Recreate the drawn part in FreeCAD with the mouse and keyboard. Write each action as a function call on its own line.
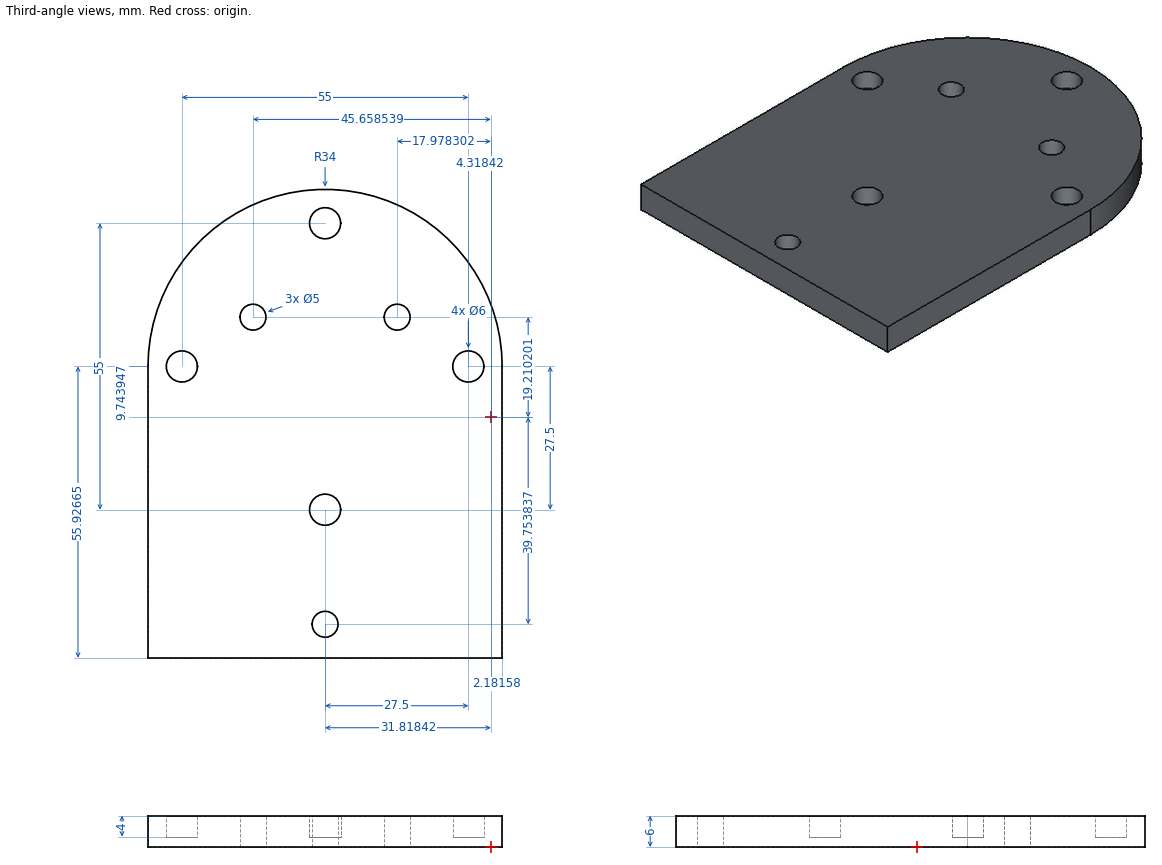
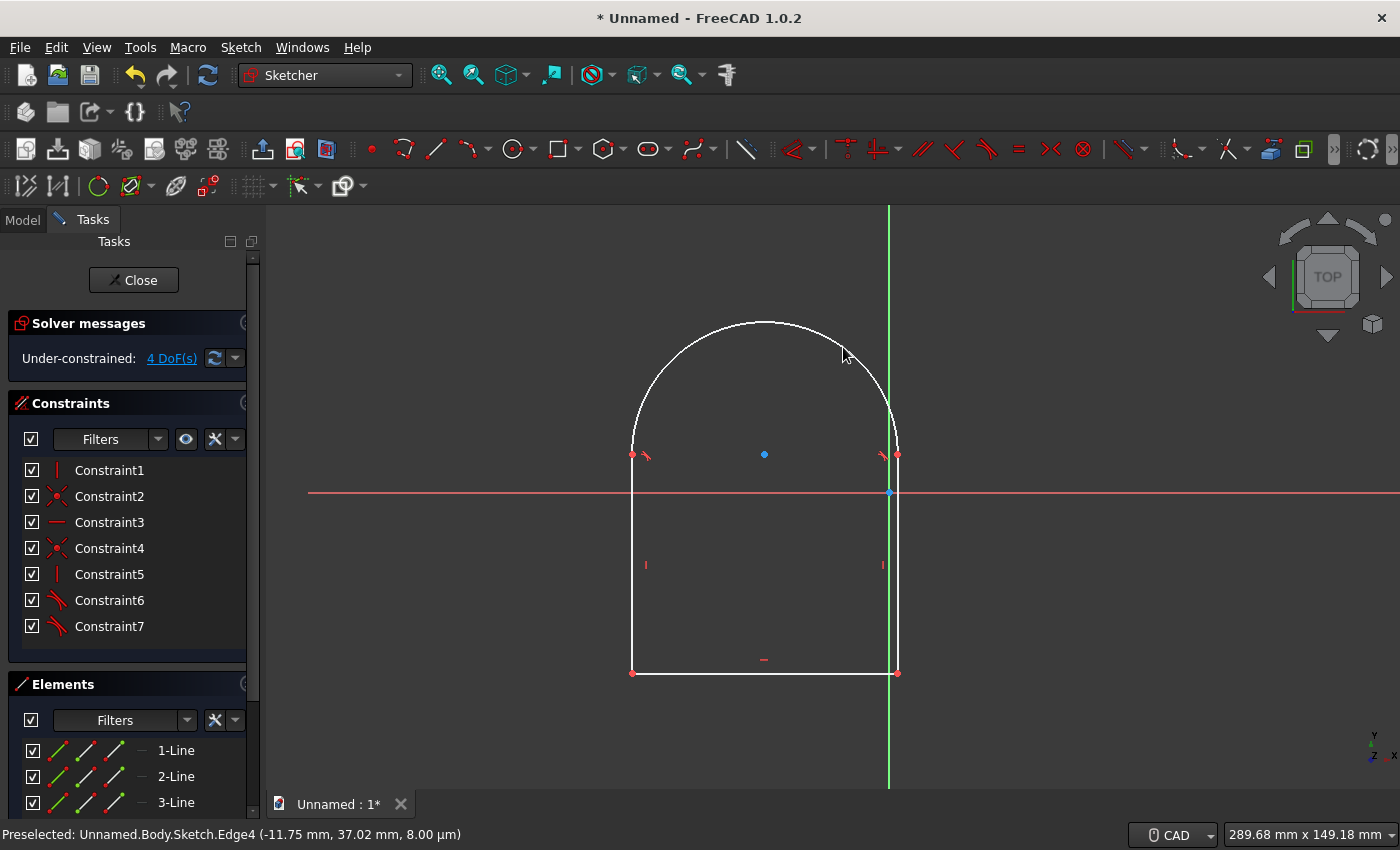
click(843, 347)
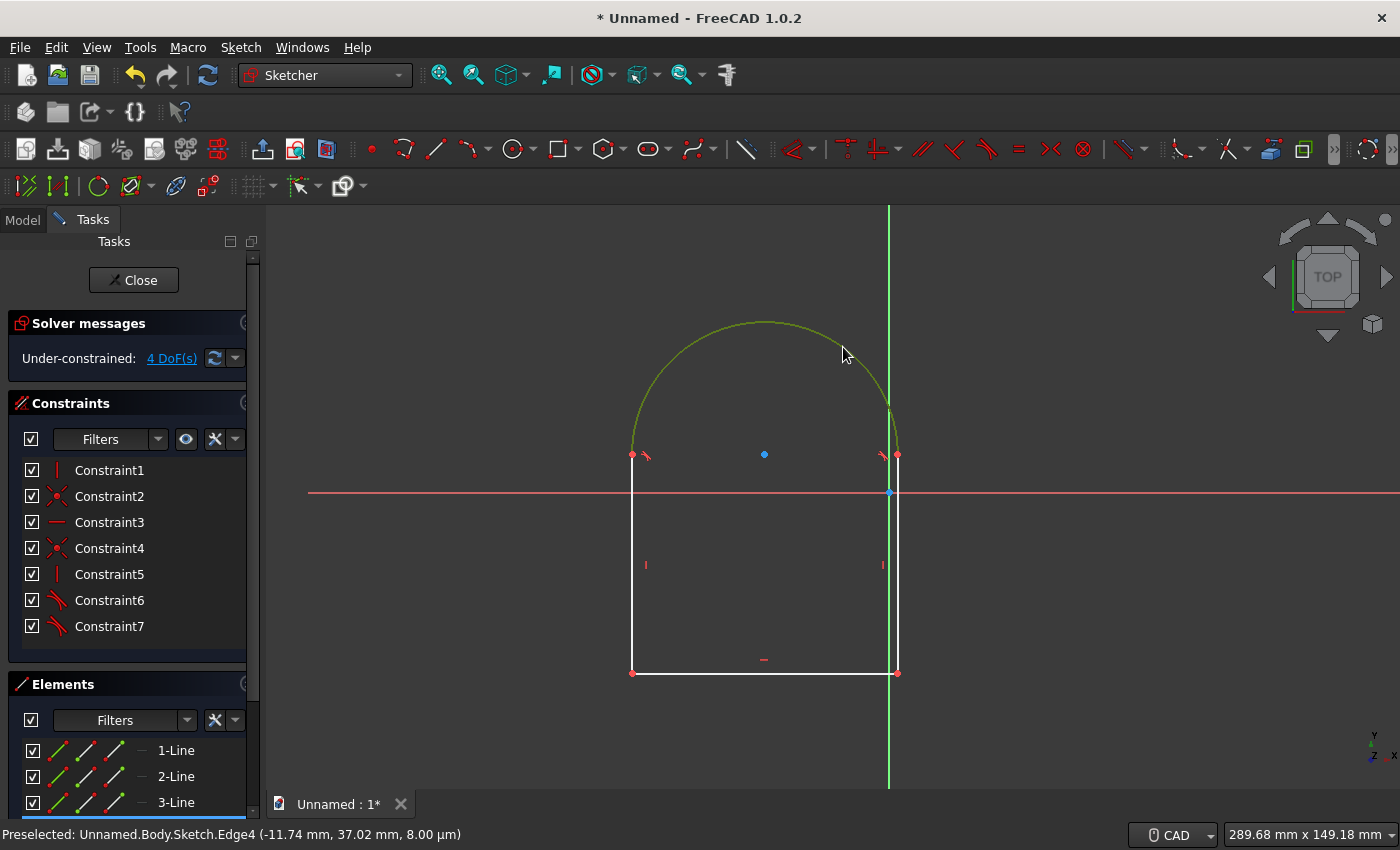
click(814, 150)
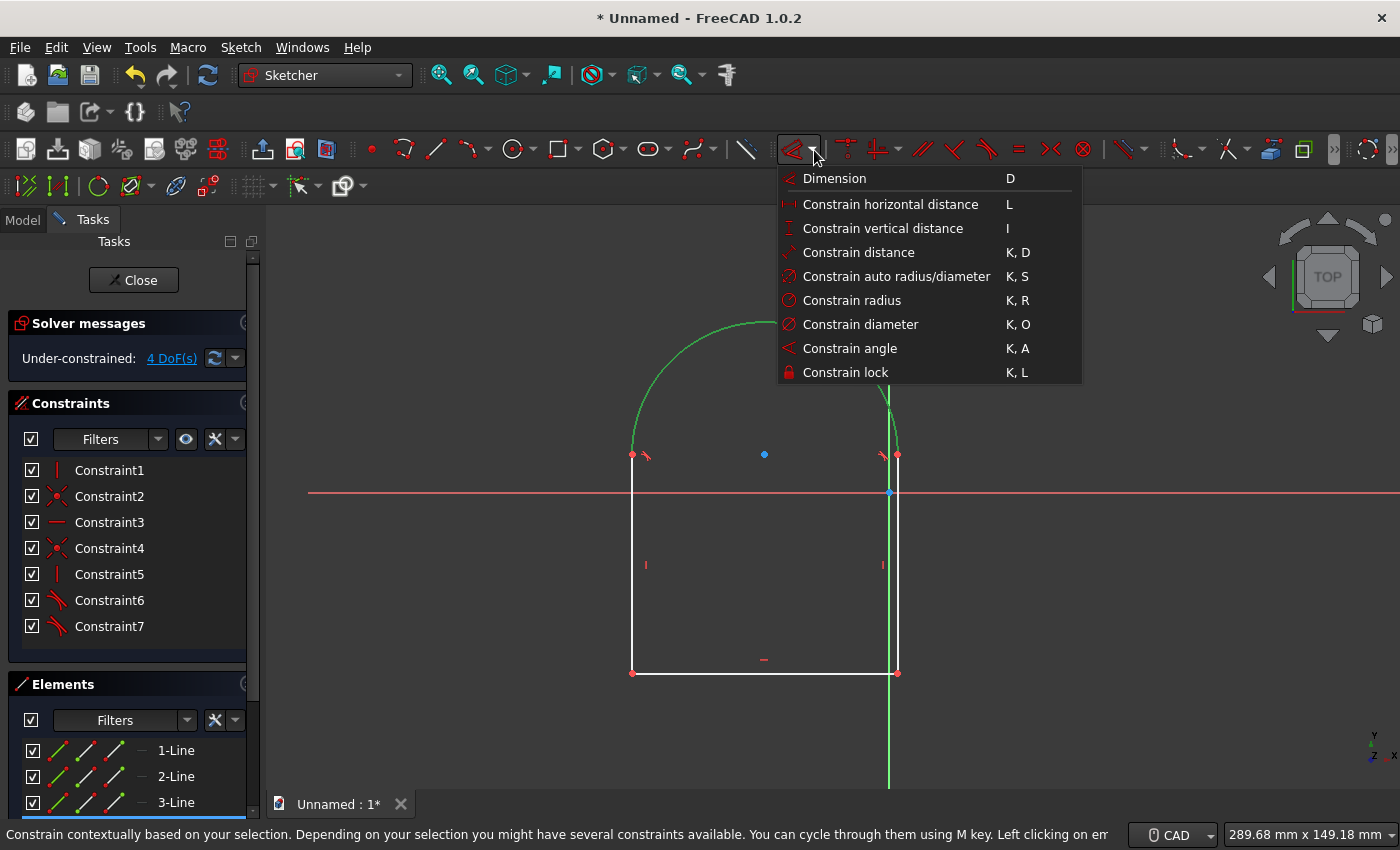
click(930, 300)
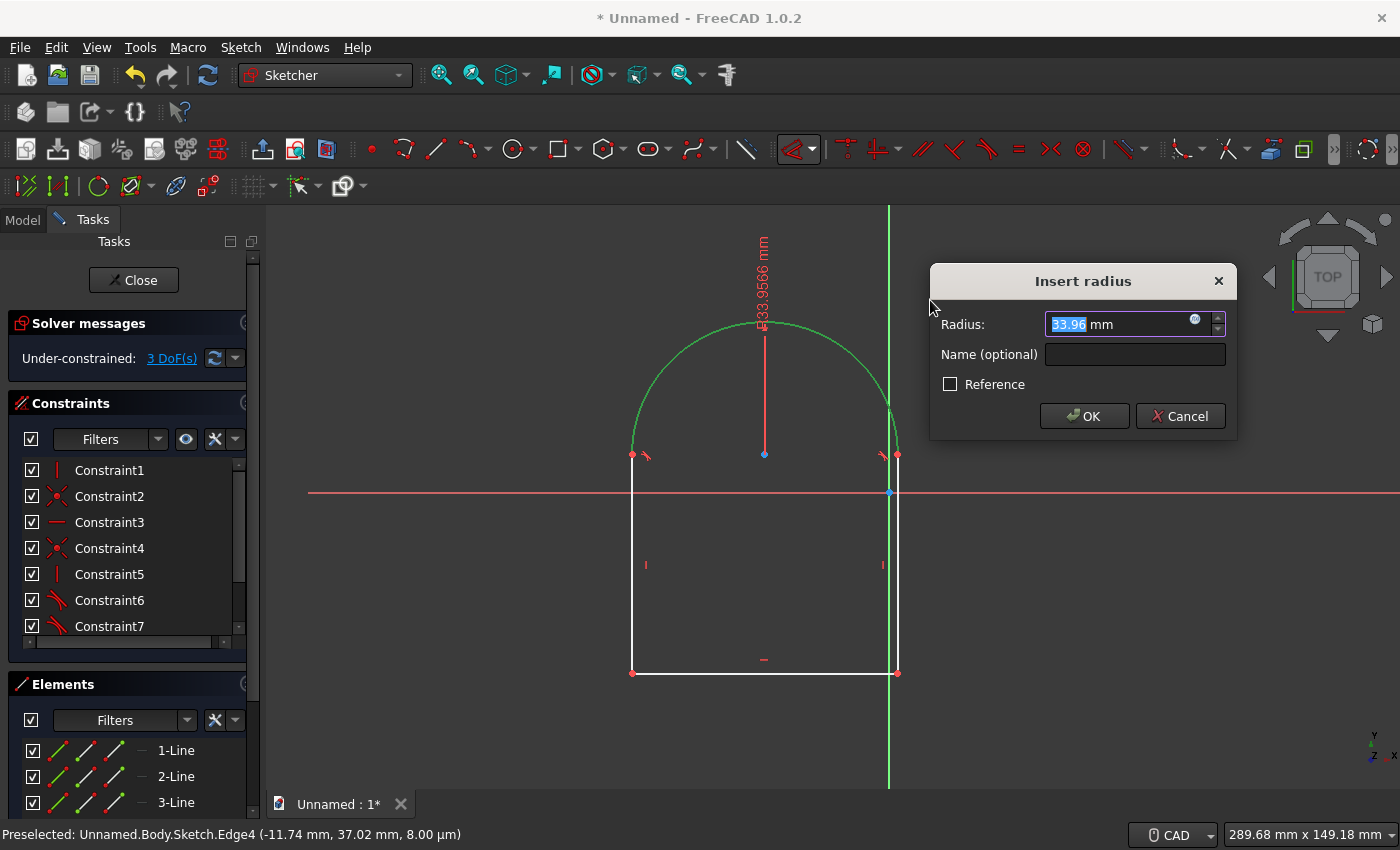
text(34)
key(Return)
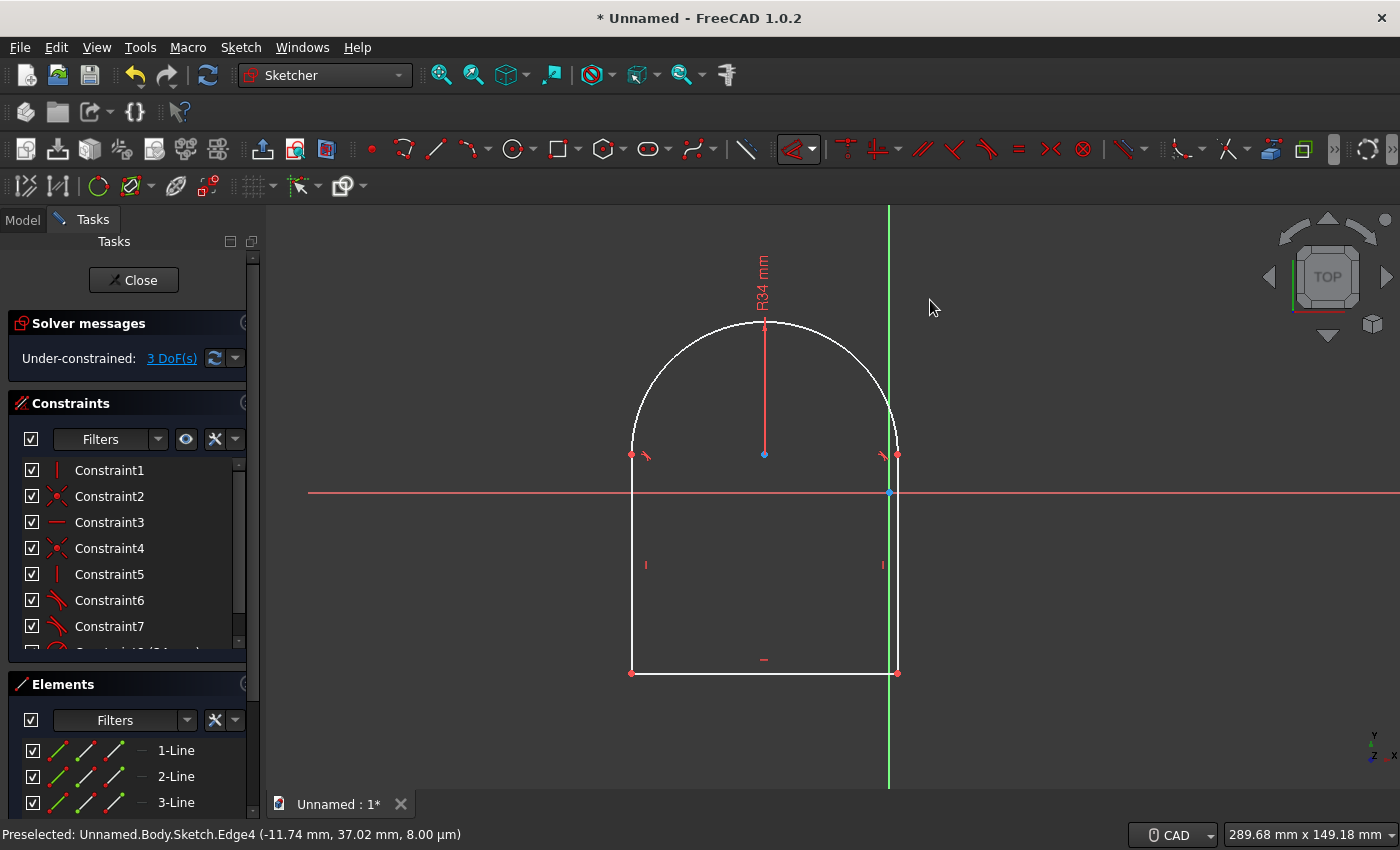
click(632, 521)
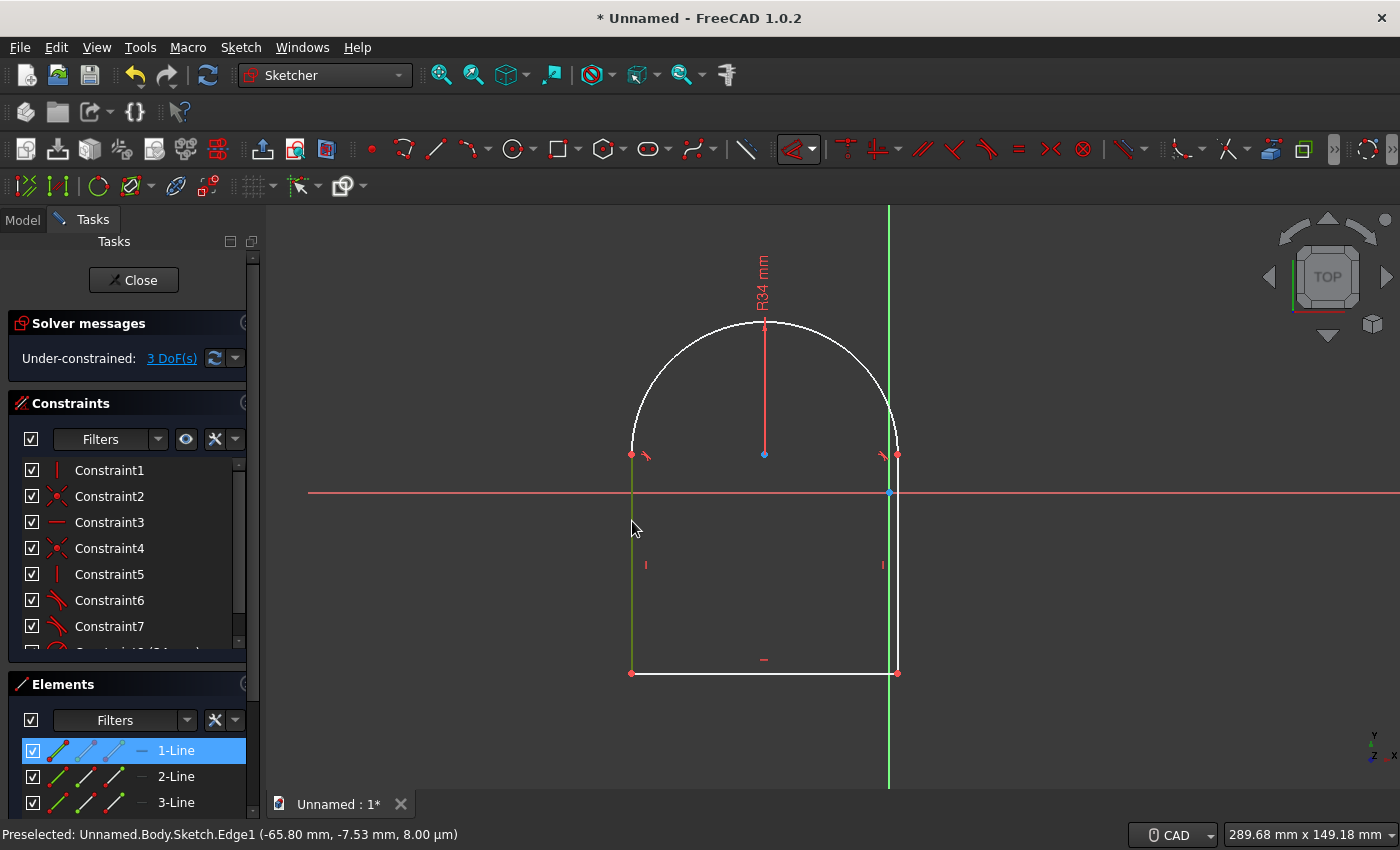
key(i)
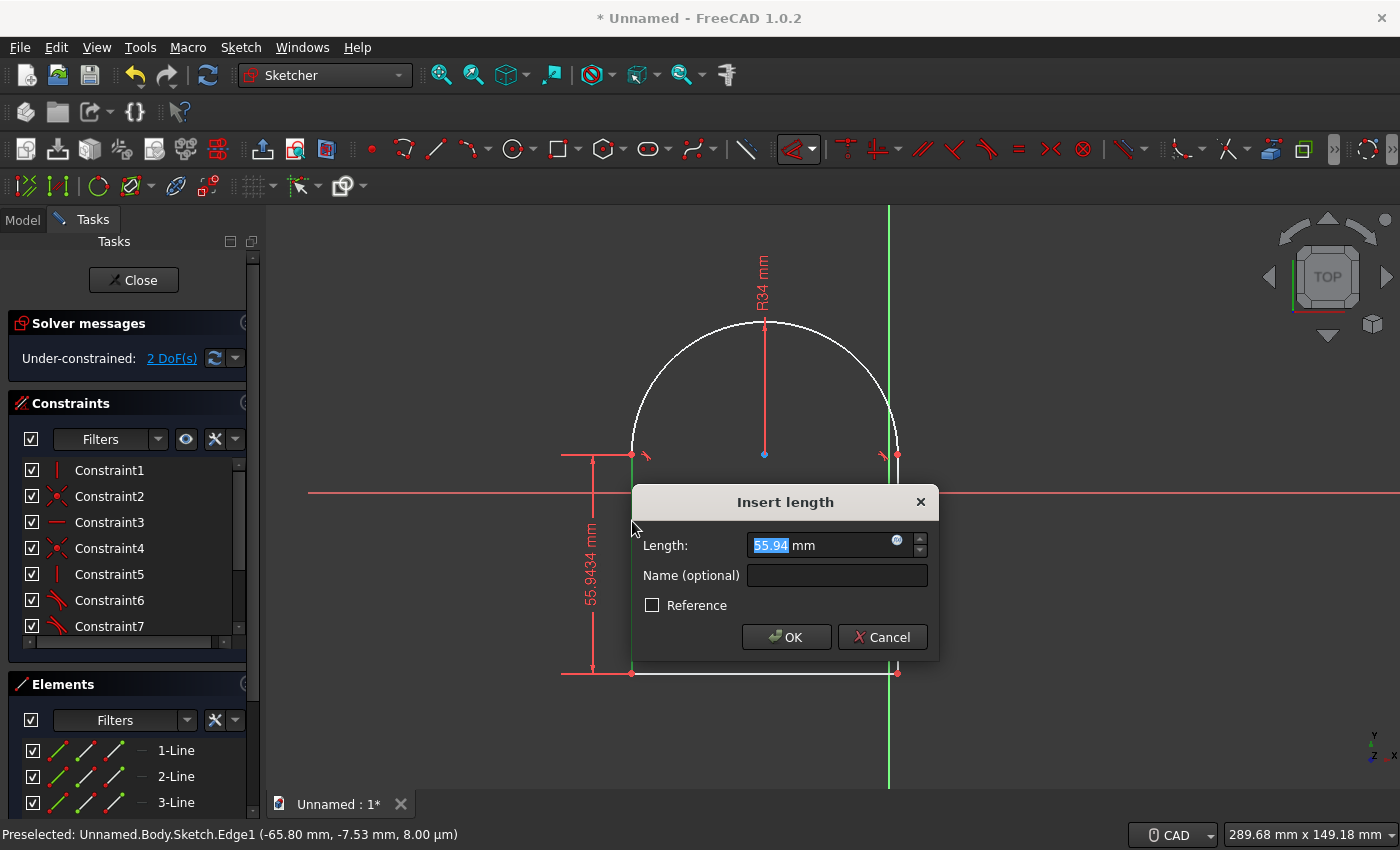
text(55.92665)
key(Return)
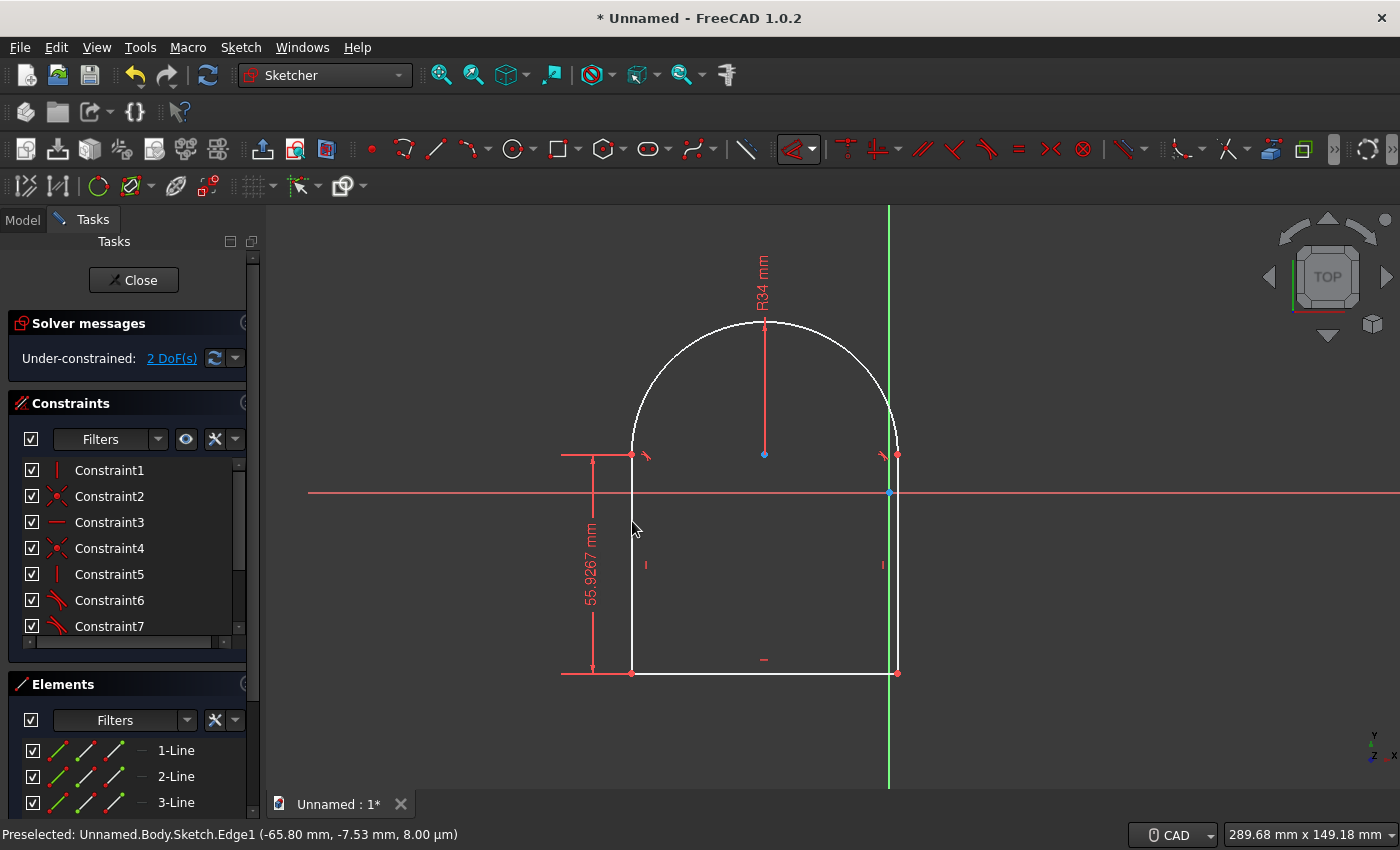
scroll(898, 674, up, 8)